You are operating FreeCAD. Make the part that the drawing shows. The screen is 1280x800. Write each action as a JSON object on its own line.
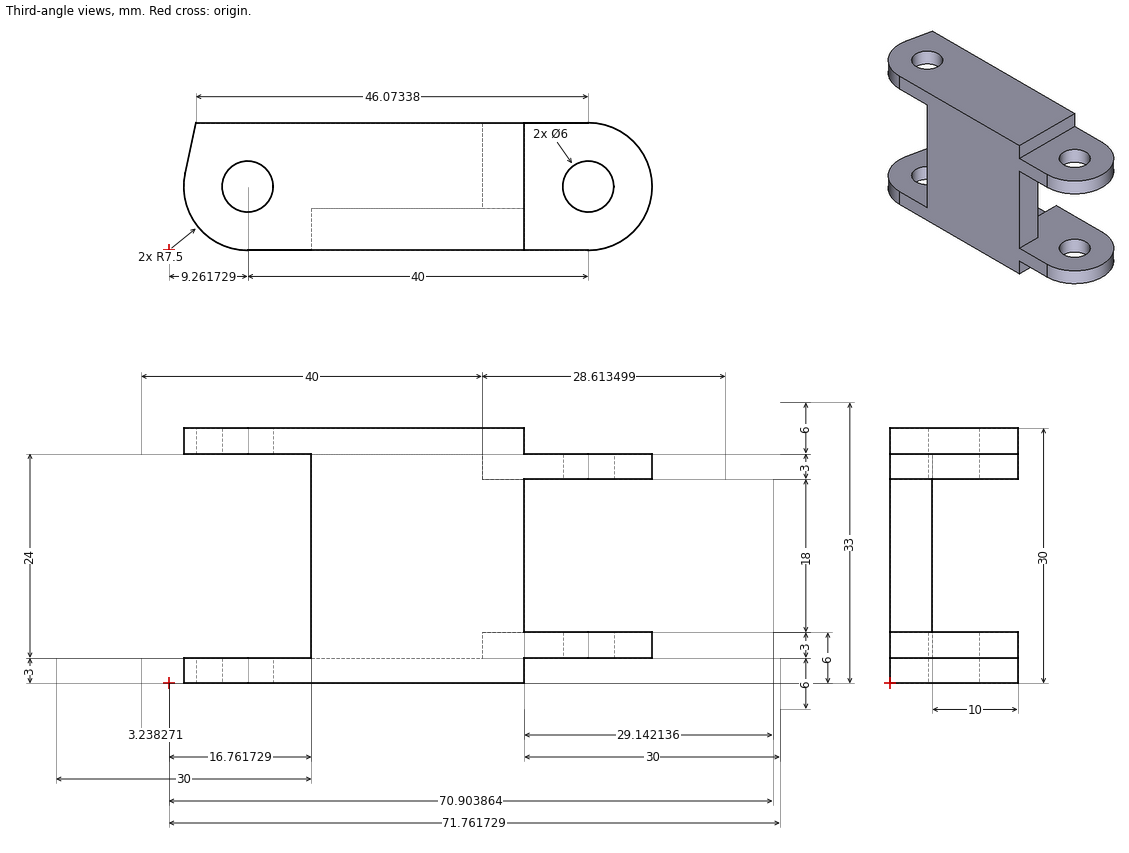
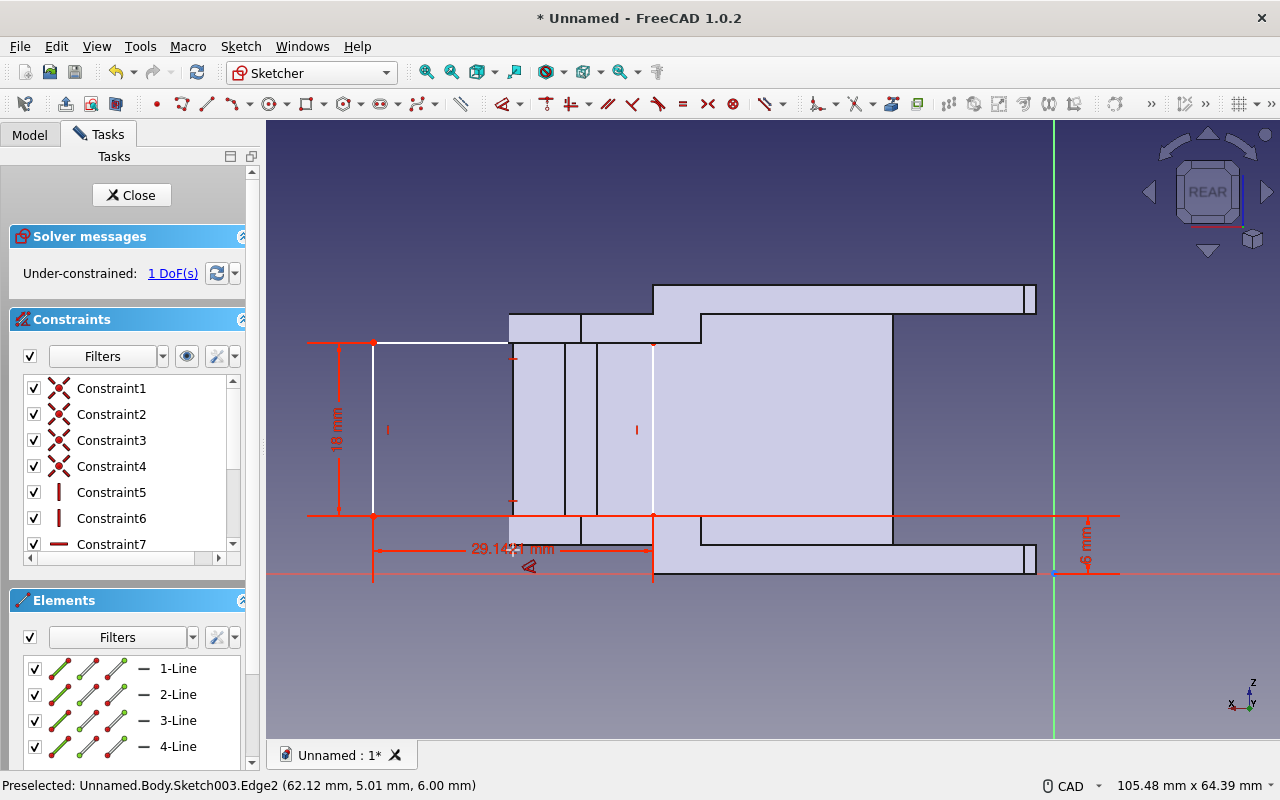
{"action": "left_click", "coordinate": [373, 343]}
{"action": "left_click", "coordinate": [714, 608]}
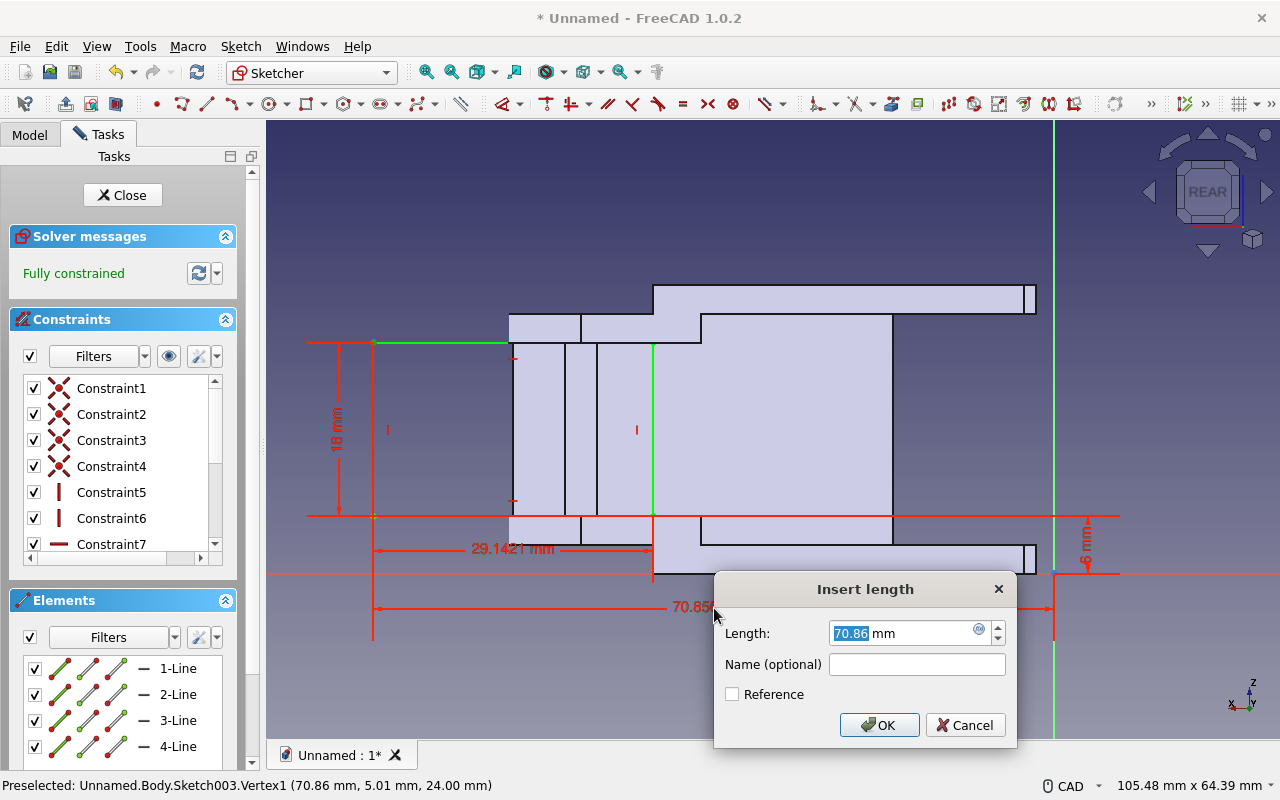
{"action": "type", "text": "70.903864"}
{"action": "key", "text": "Return"}
{"action": "key", "text": "Escape"}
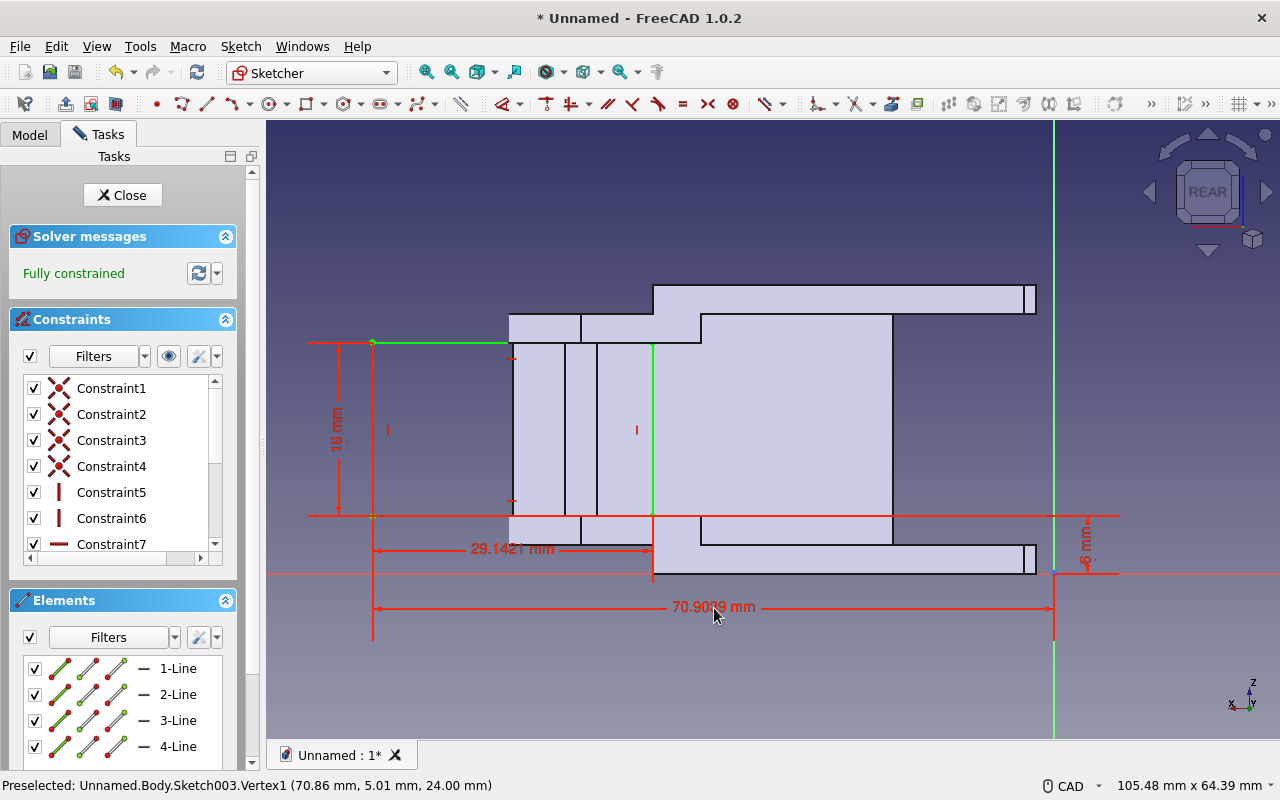
{"action": "left_click", "coordinate": [123, 195]}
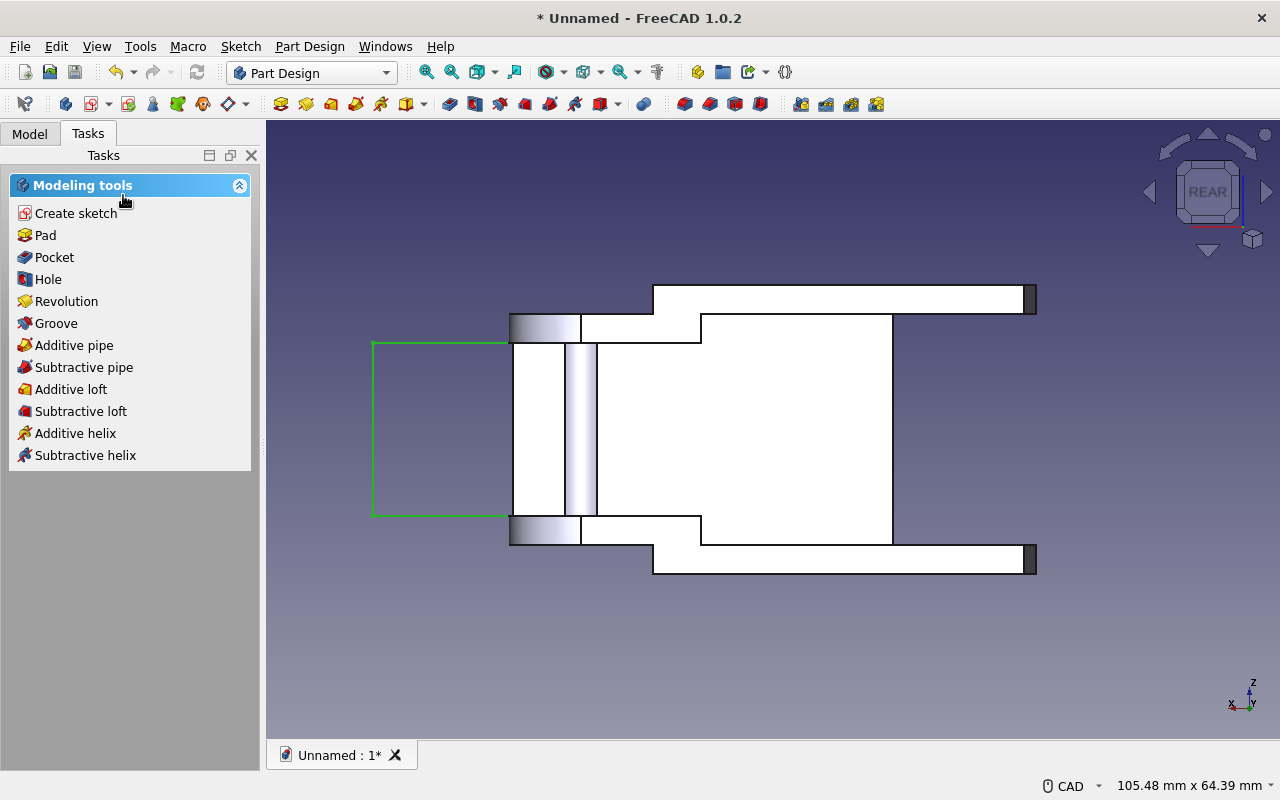
{"action": "left_click", "coordinate": [450, 104]}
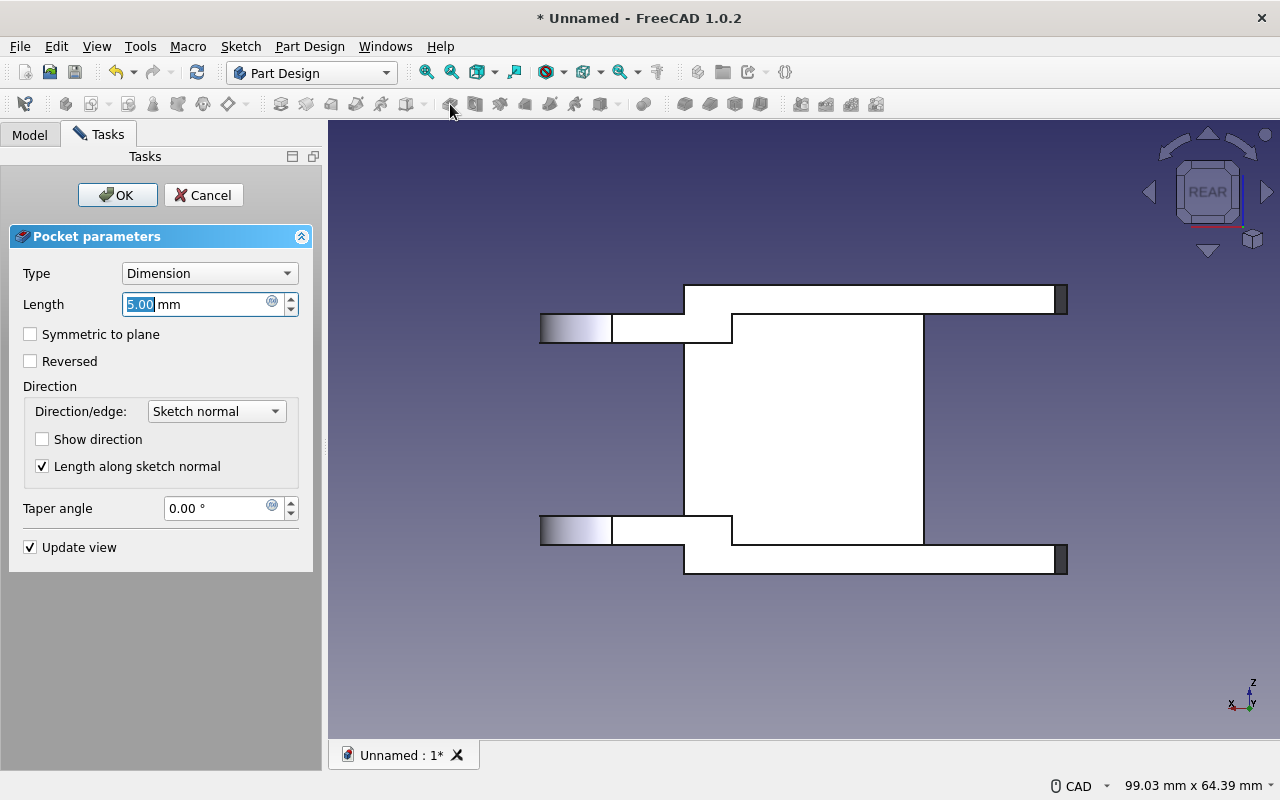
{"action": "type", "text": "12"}
{"action": "key", "text": "Tab"}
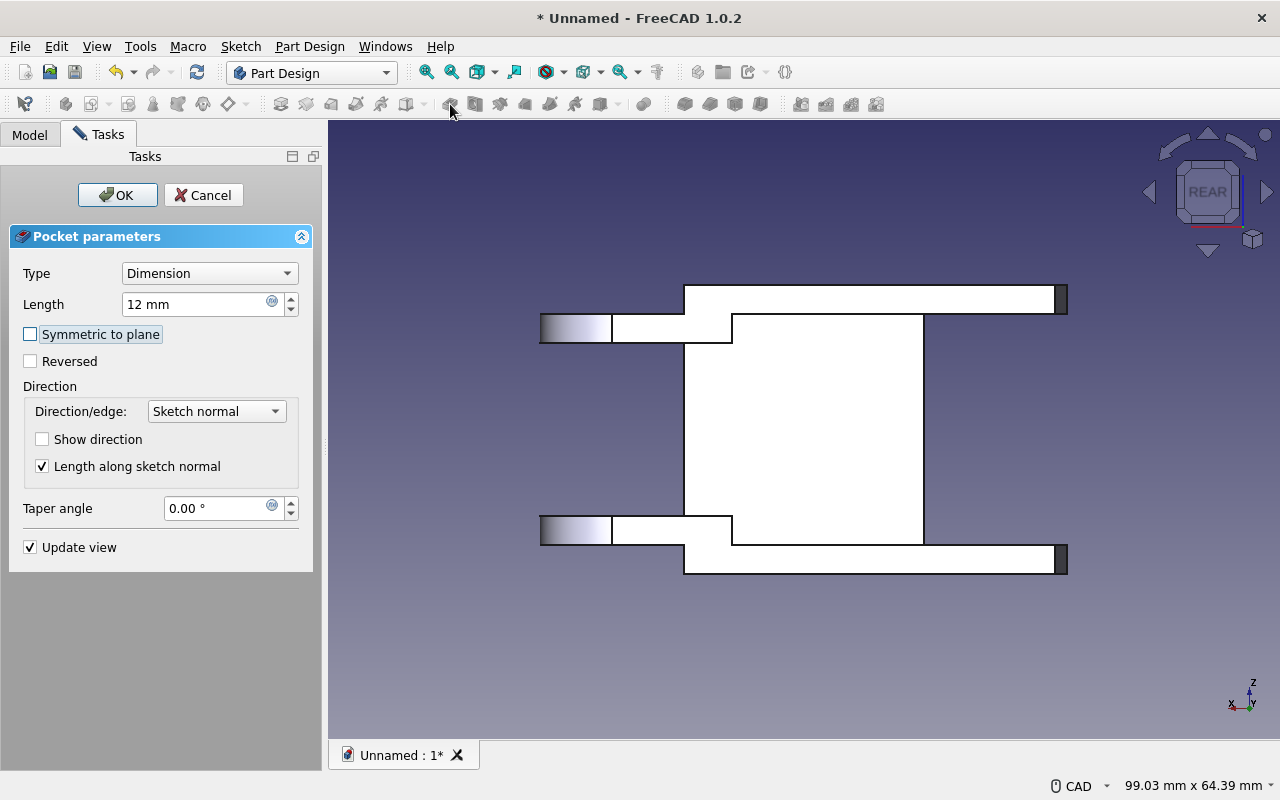
{"action": "left_click", "coordinate": [118, 195]}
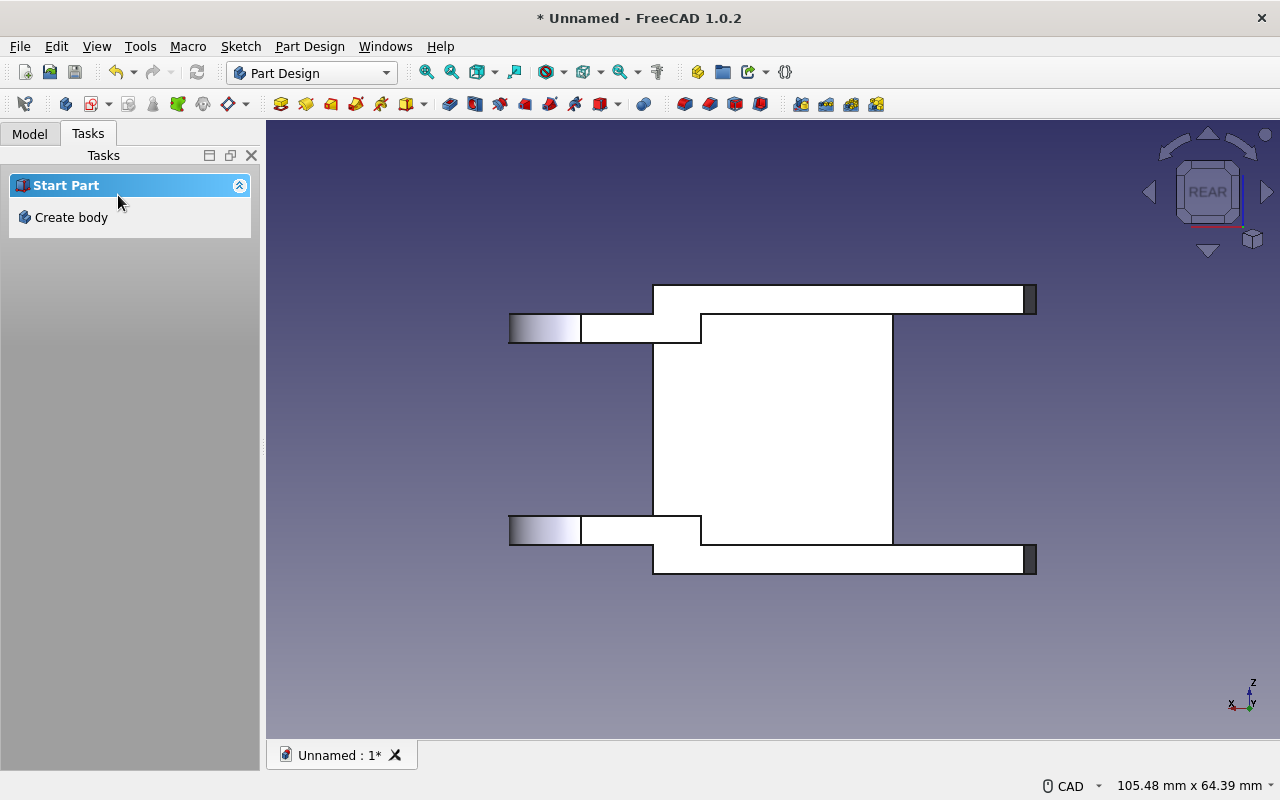
{"action": "key", "text": "0"}